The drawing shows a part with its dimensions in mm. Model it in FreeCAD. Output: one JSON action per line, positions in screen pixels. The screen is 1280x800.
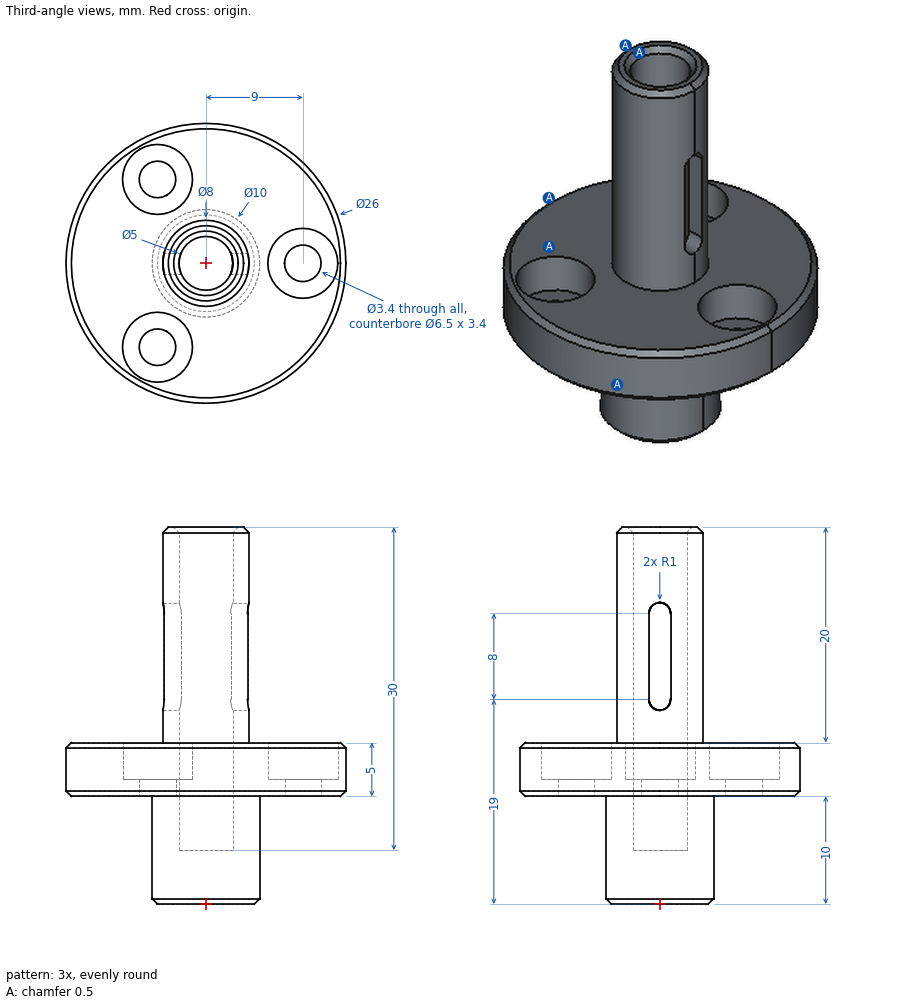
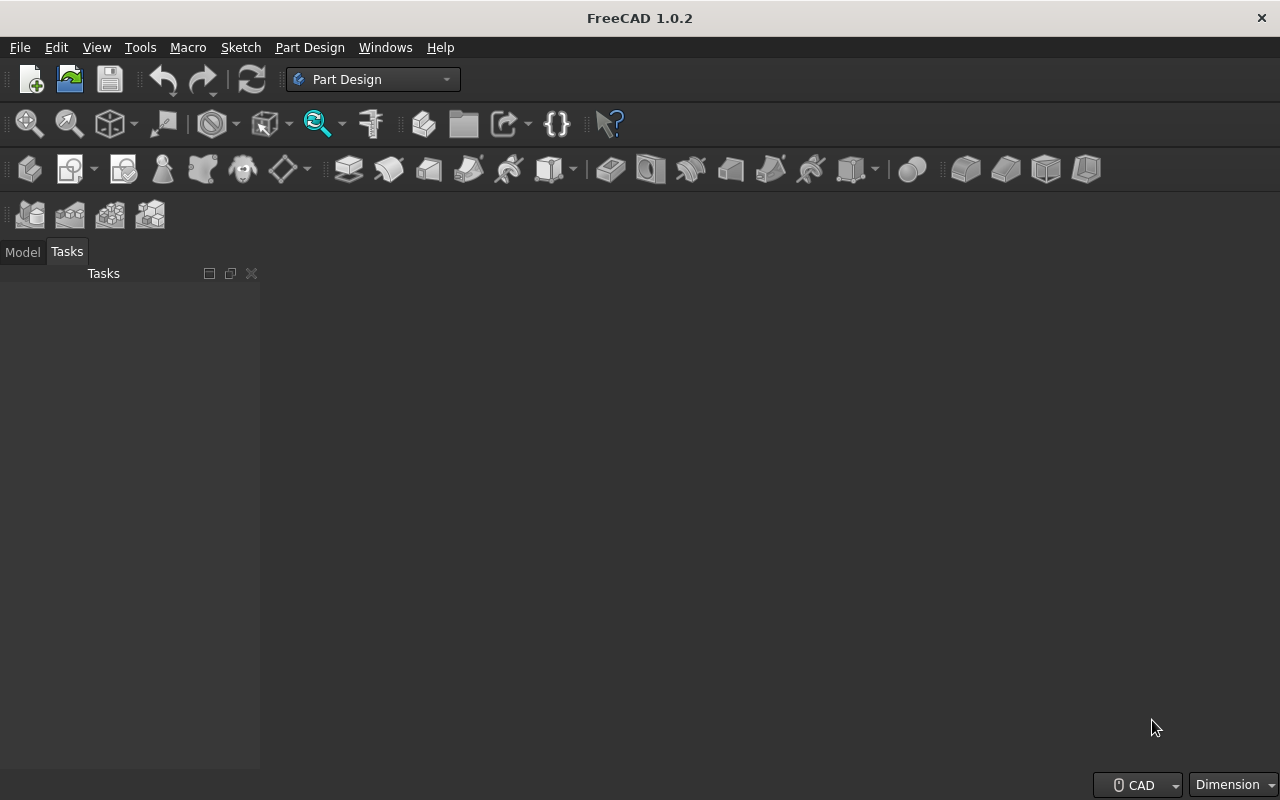
{"action": "left_click", "coordinate": [30, 80]}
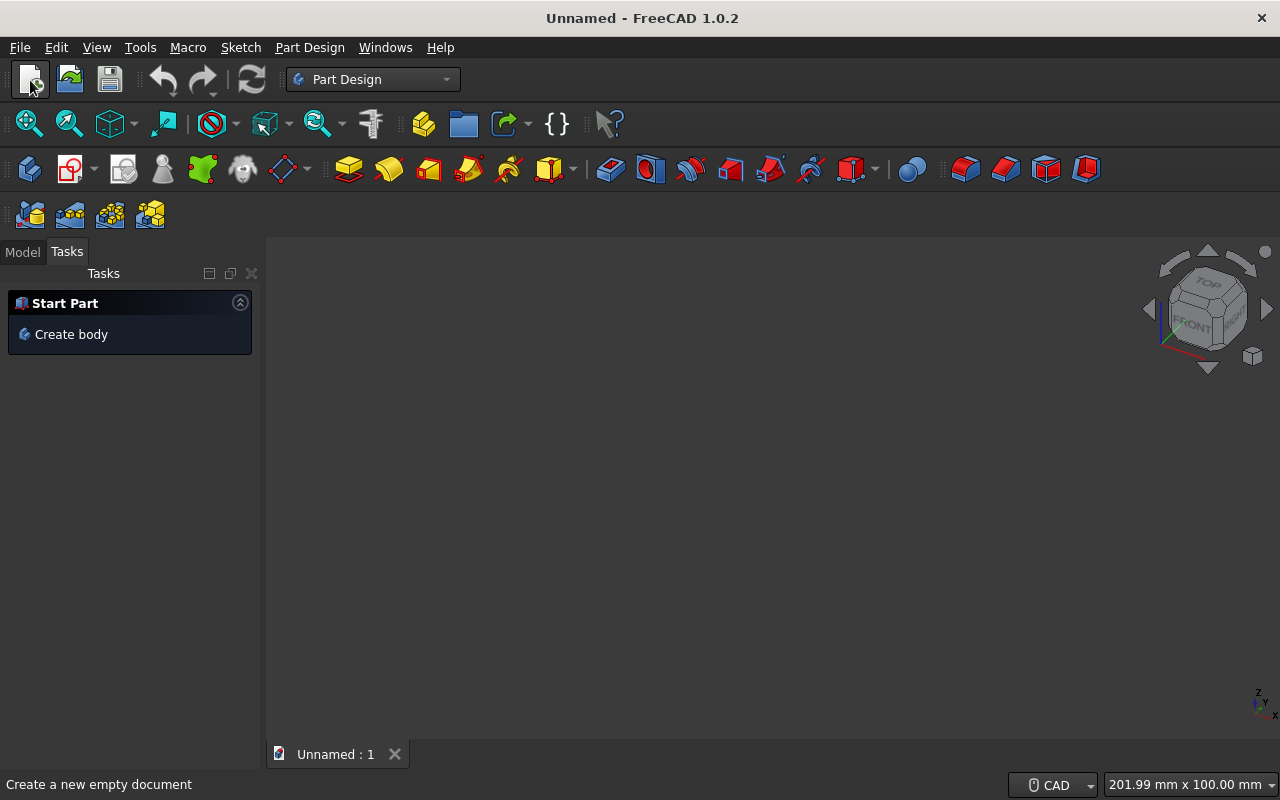
{"action": "left_click", "coordinate": [70, 170]}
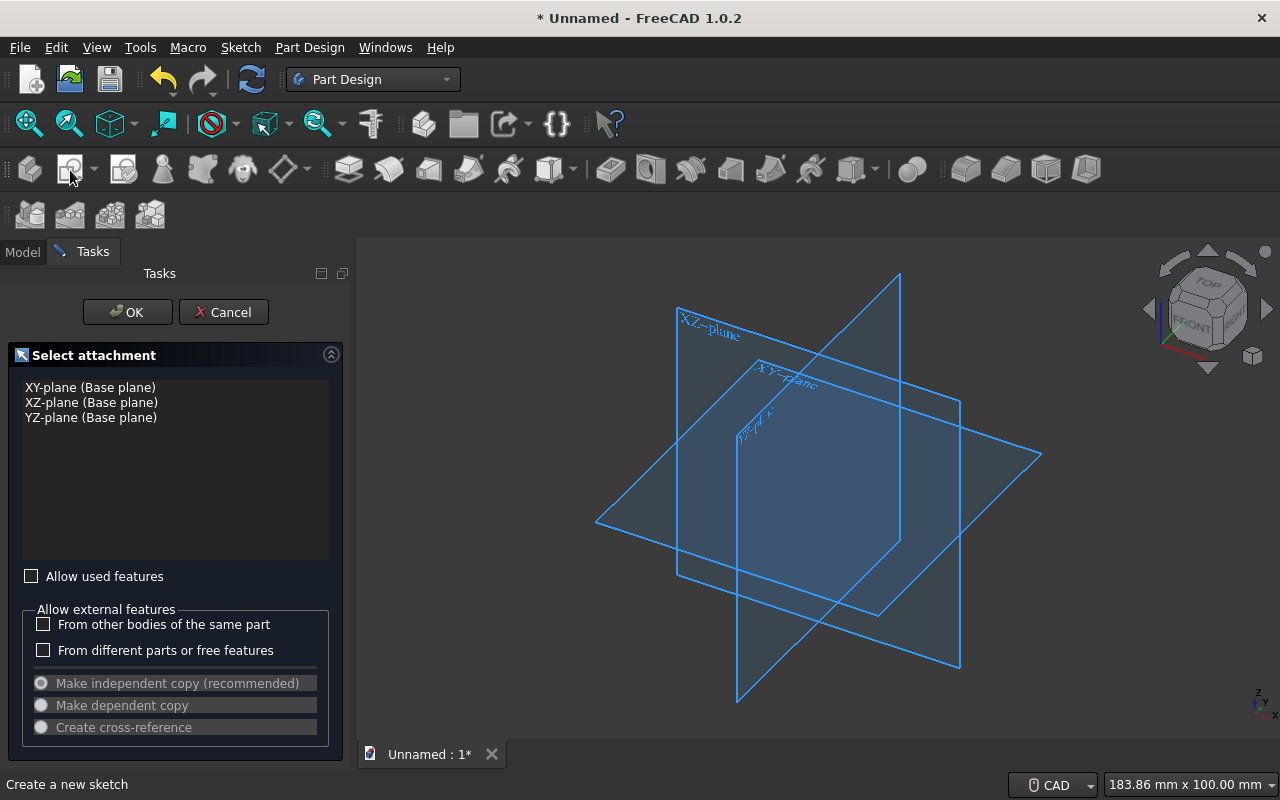
{"action": "left_click", "coordinate": [82, 388]}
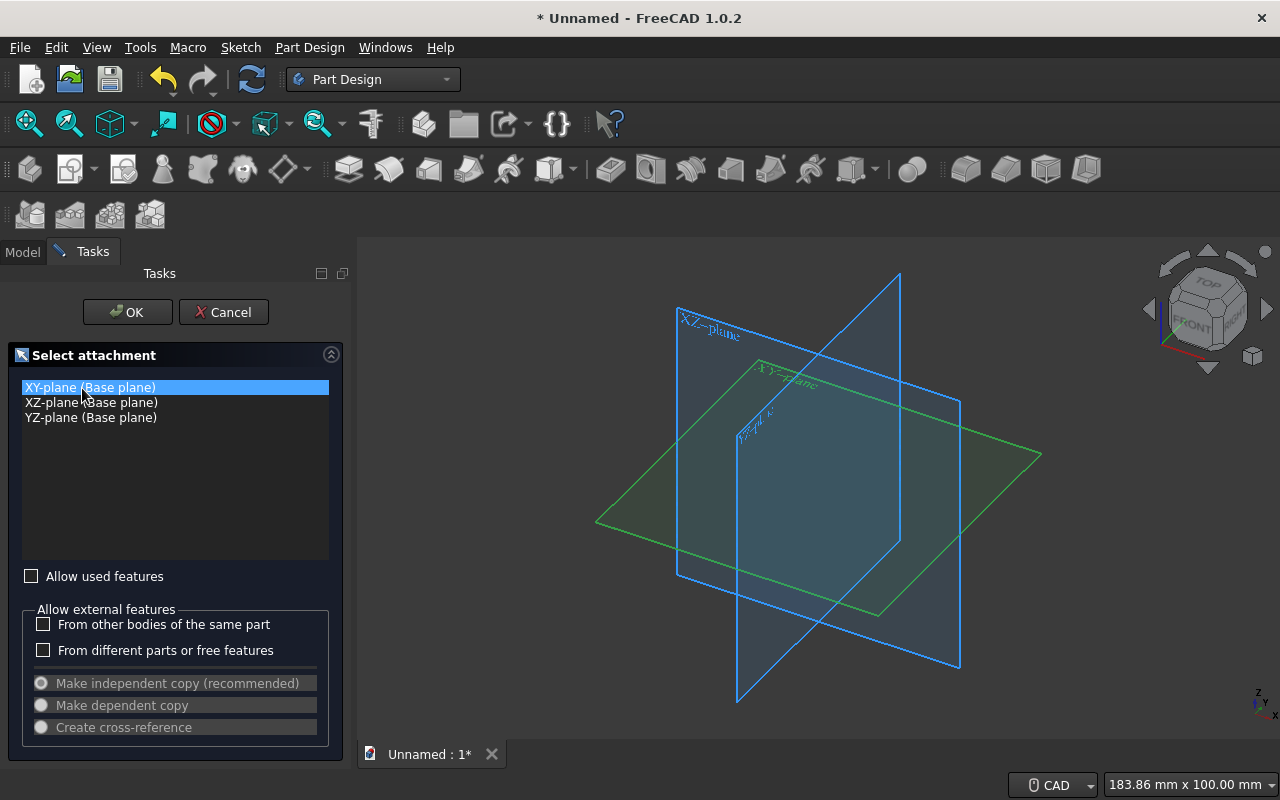
{"action": "left_click", "coordinate": [128, 312]}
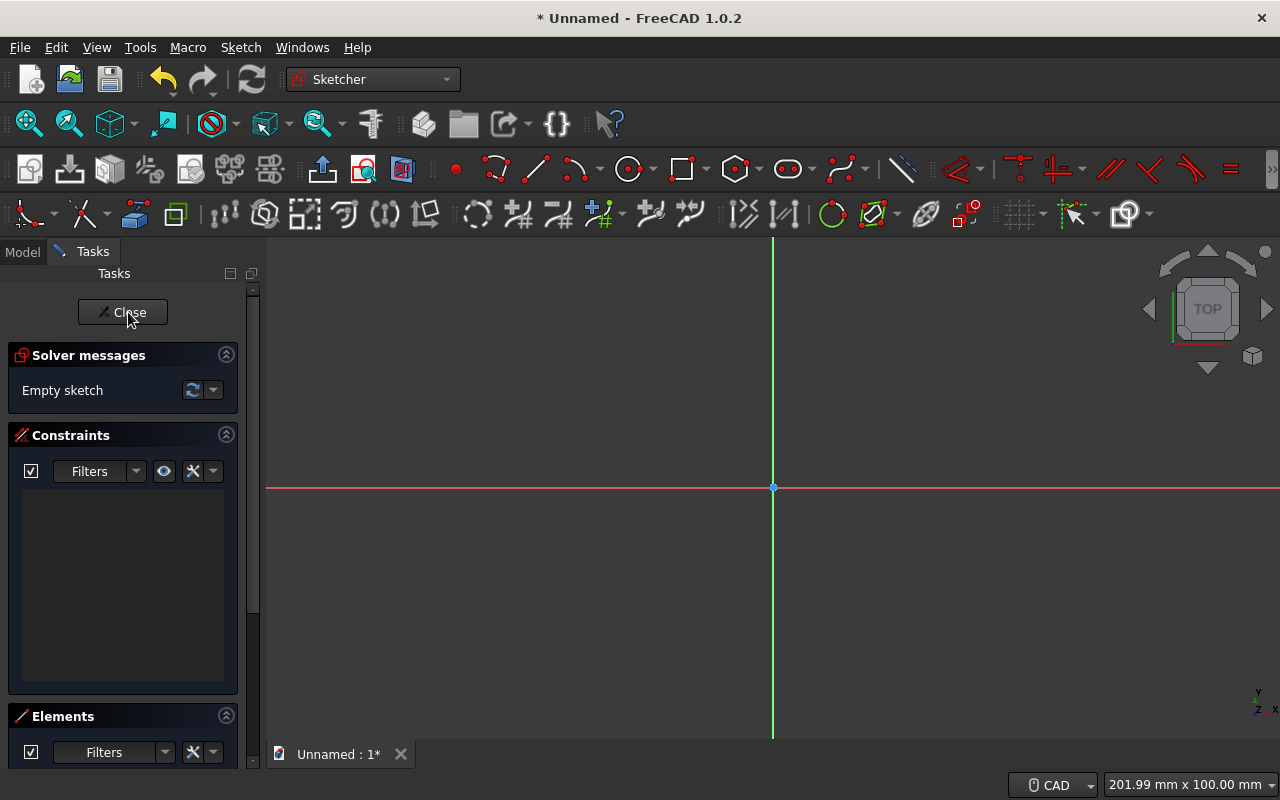
{"action": "scroll", "coordinate": [787, 488], "scroll_direction": "up", "scroll_amount": 9}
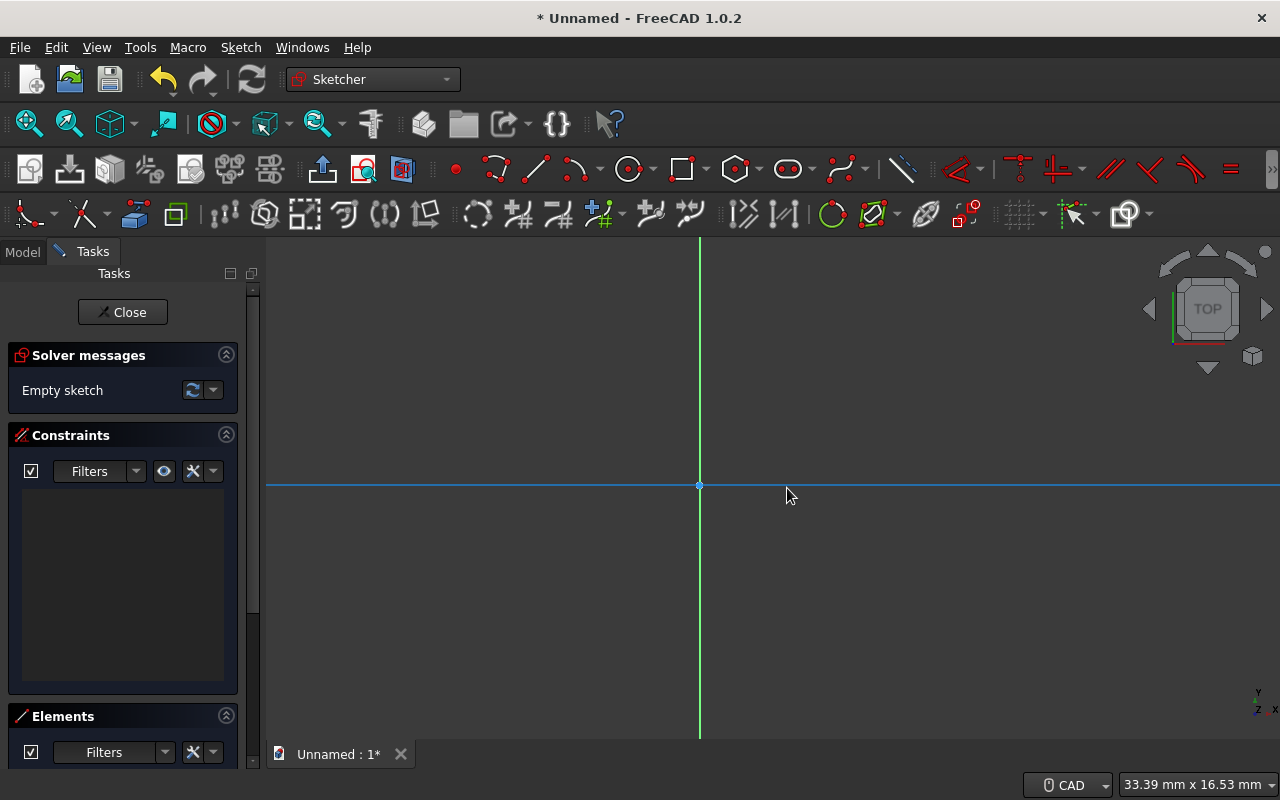
{"action": "left_click", "coordinate": [630, 170]}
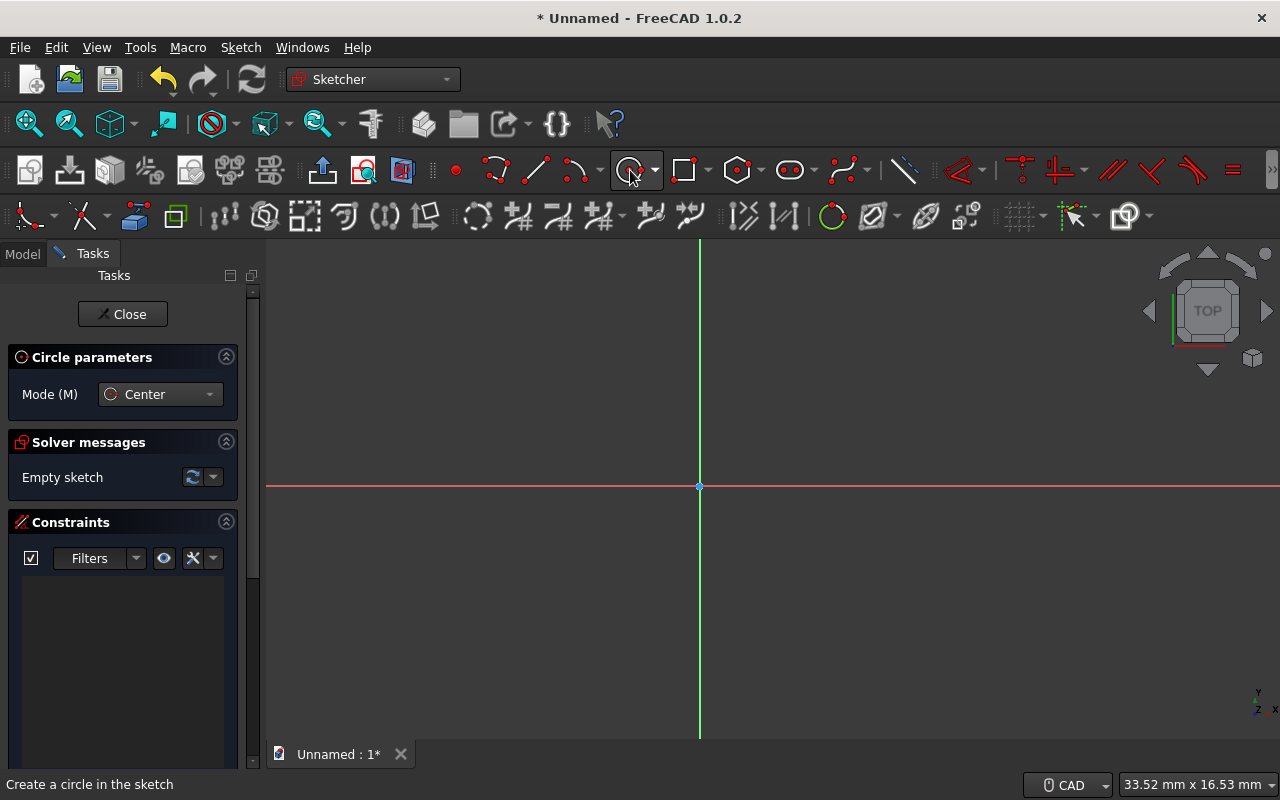
{"action": "left_click", "coordinate": [700, 486]}
{"action": "left_click", "coordinate": [807, 380]}
{"action": "key", "text": "Escape"}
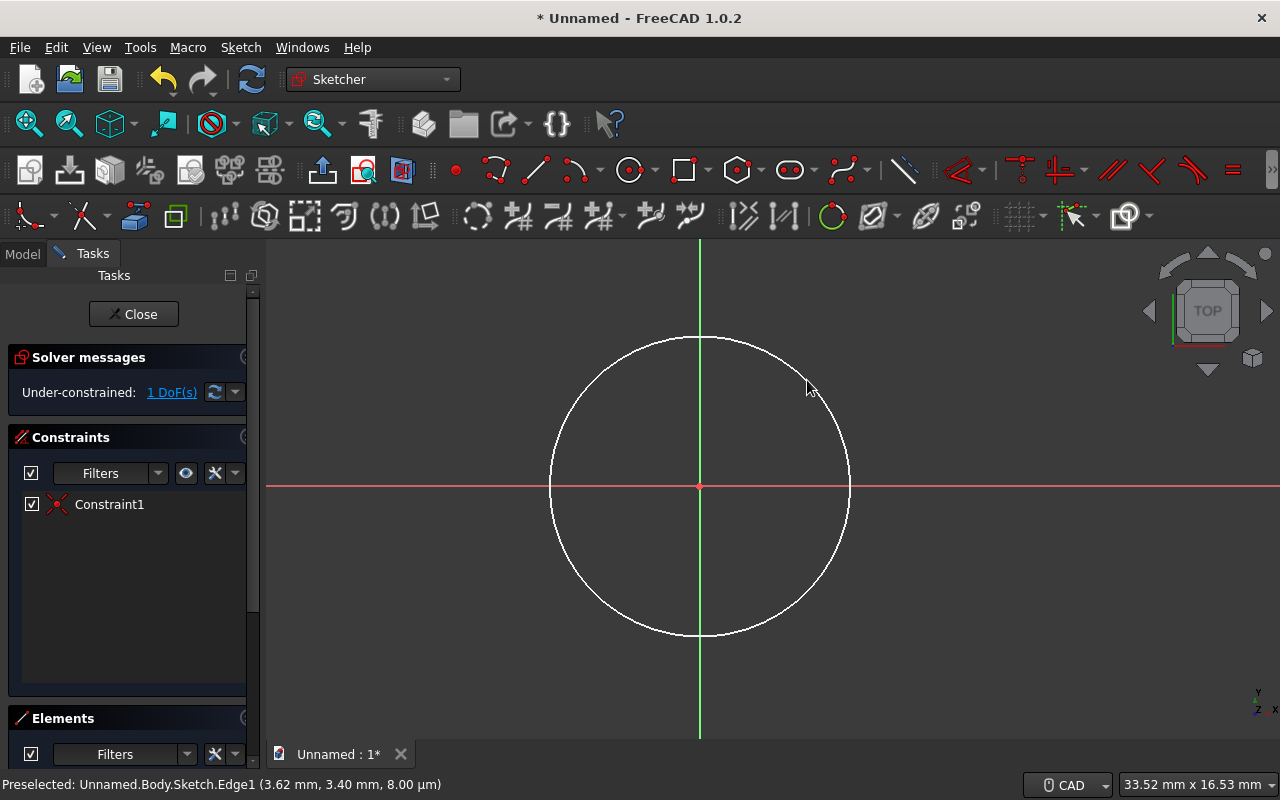
{"action": "left_click", "coordinate": [806, 380]}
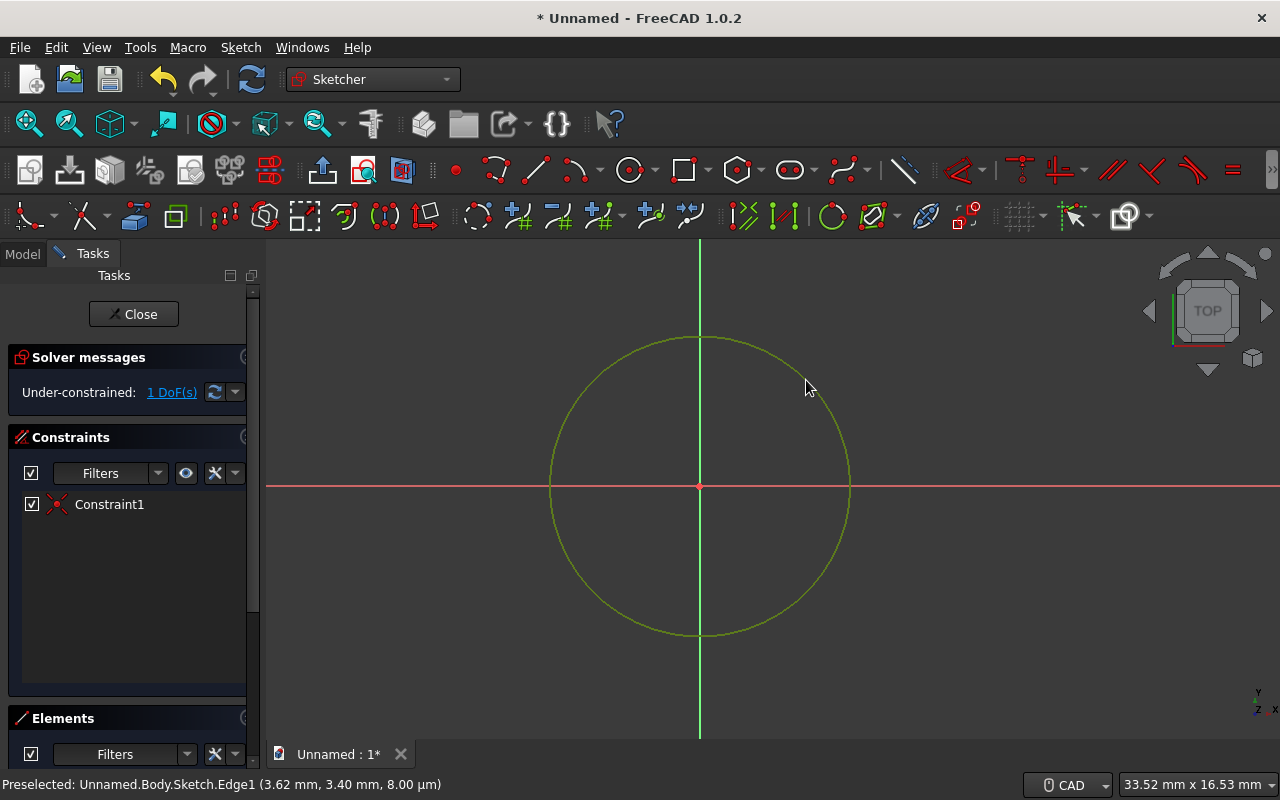
{"action": "left_click", "coordinate": [984, 170]}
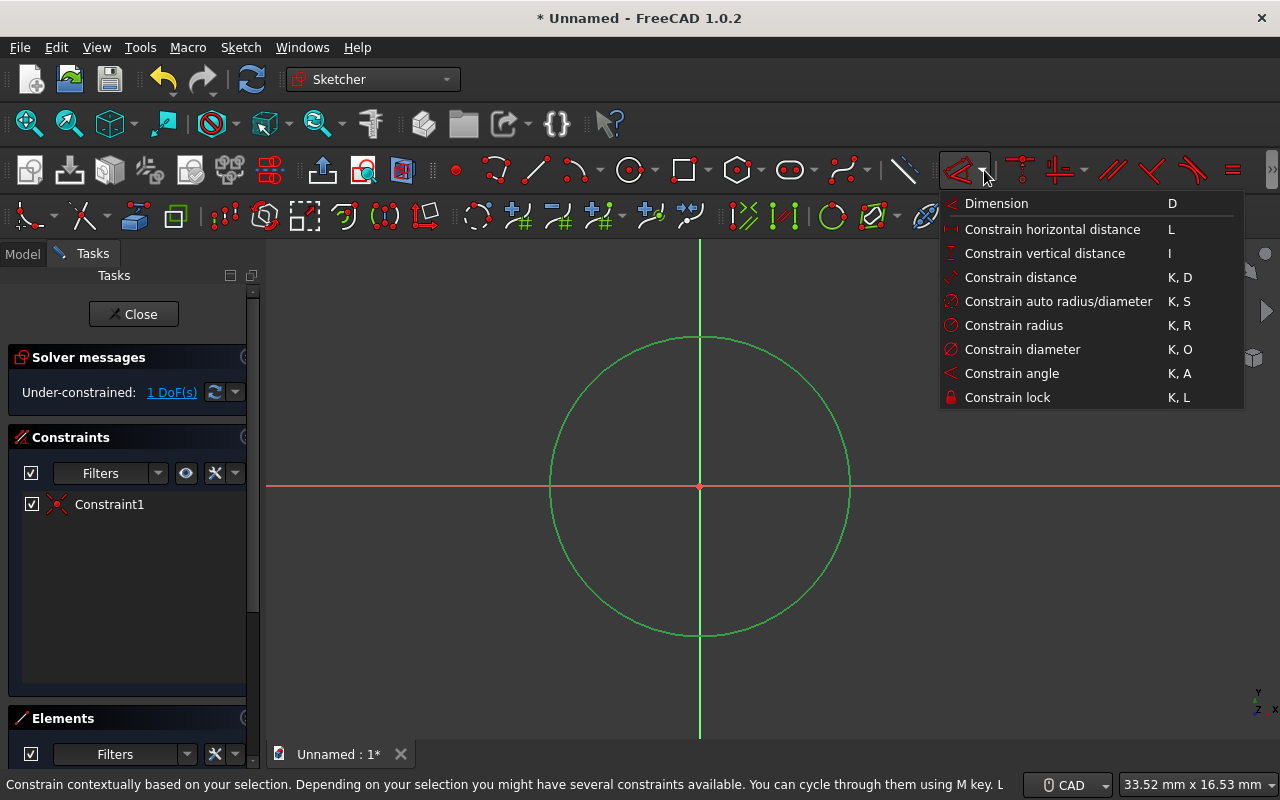
{"action": "left_click", "coordinate": [1092, 349]}